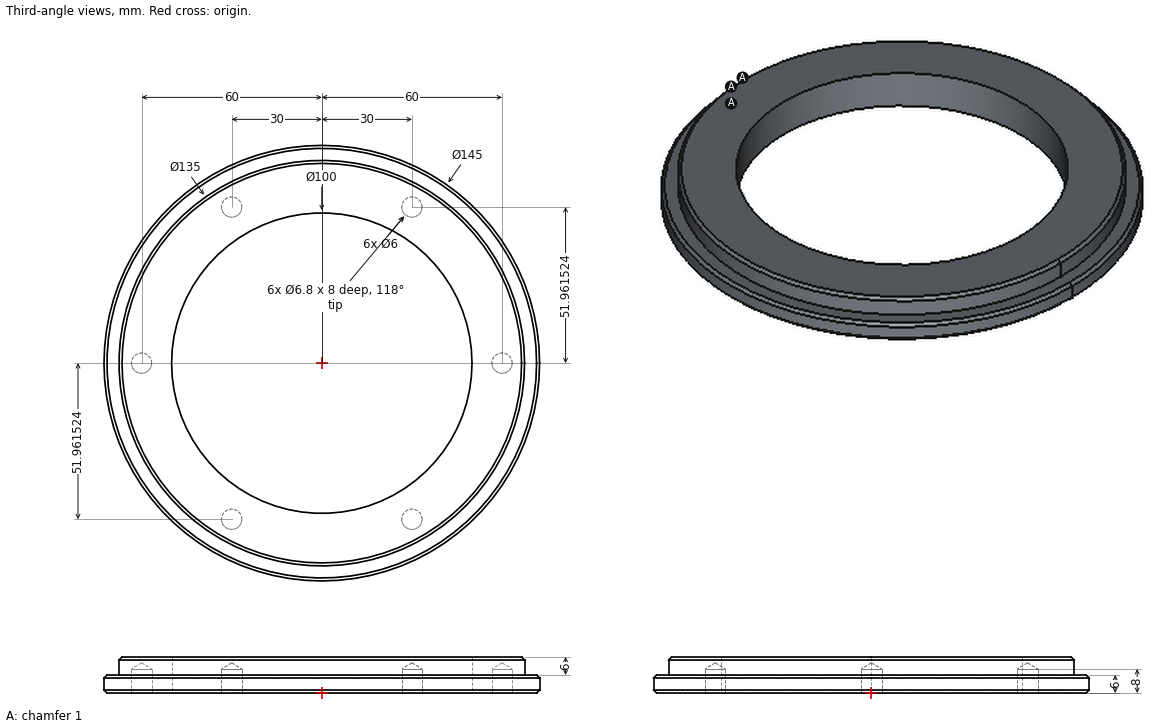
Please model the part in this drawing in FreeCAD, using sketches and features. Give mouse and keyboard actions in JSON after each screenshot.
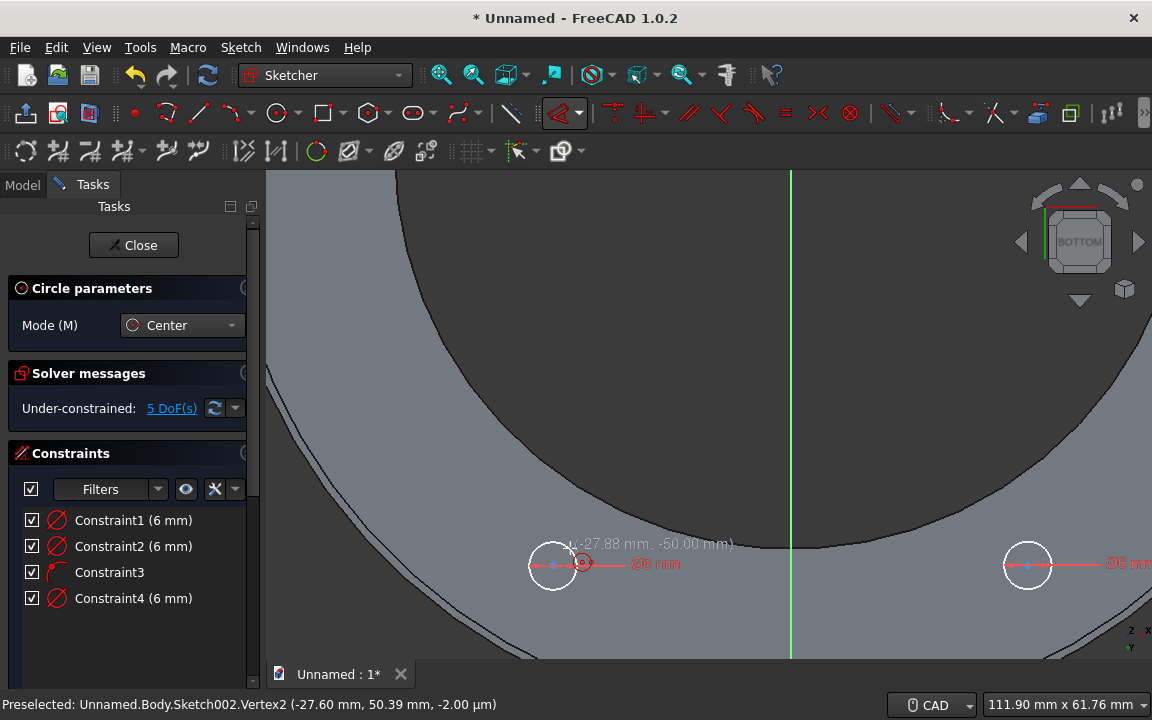
{"action": "scroll", "coordinate": [553, 567], "scroll_direction": "down", "scroll_amount": 5}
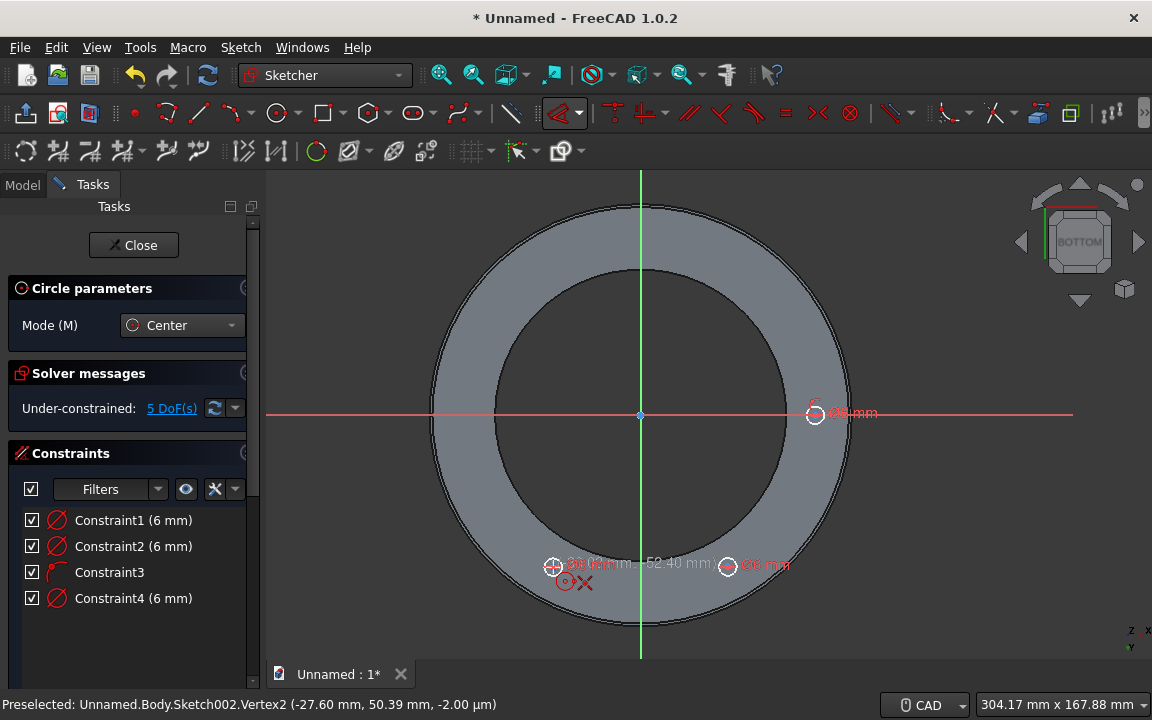
{"action": "scroll", "coordinate": [466, 415], "scroll_direction": "up", "scroll_amount": 5}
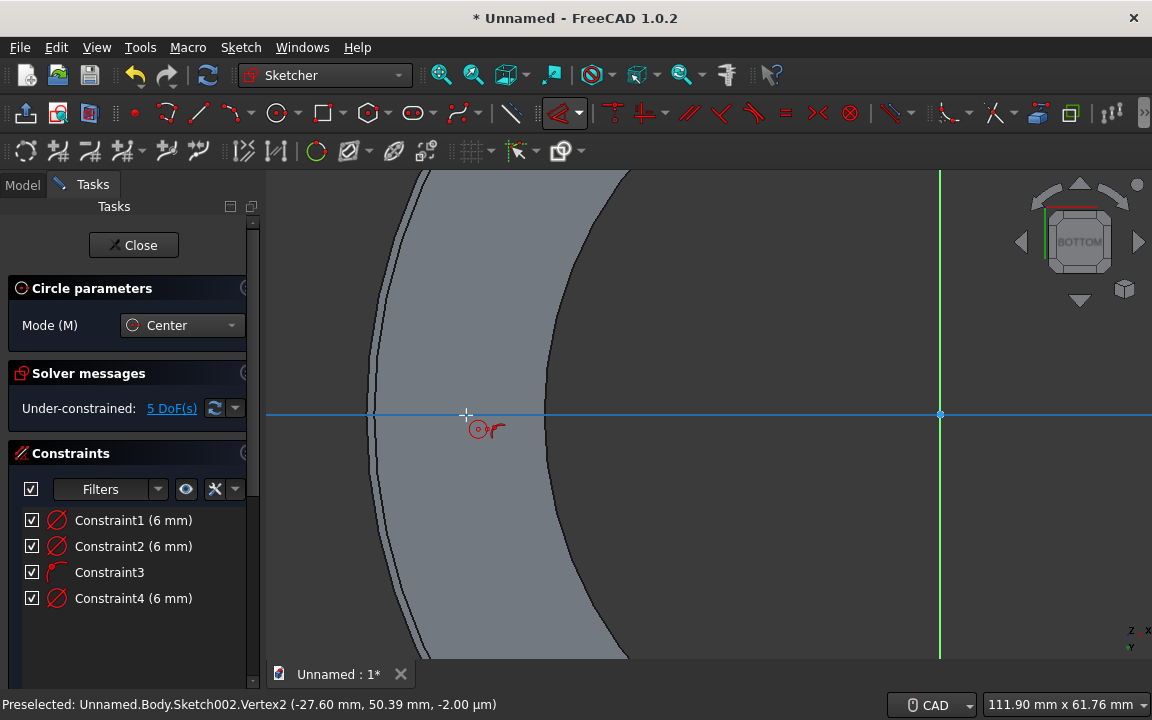
{"action": "left_click", "coordinate": [465, 415]}
{"action": "mouse_move", "coordinate": [482, 398]}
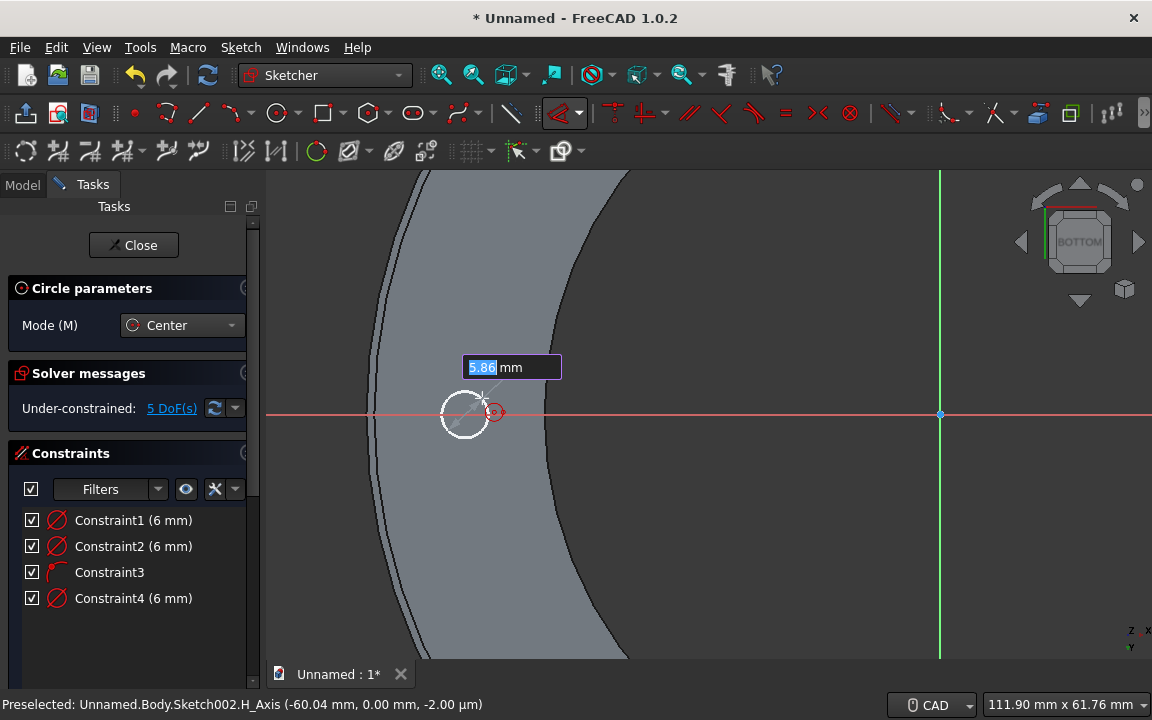
{"action": "type", "text": "6"}
{"action": "key", "text": "Return"}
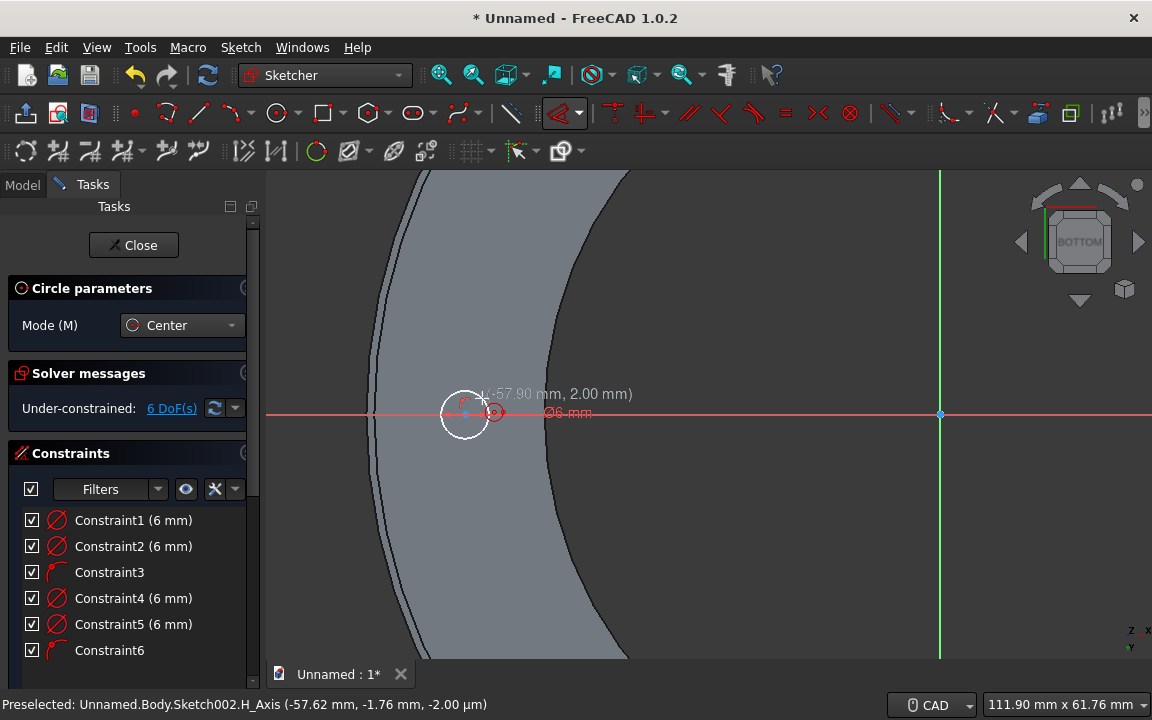
{"action": "scroll", "coordinate": [466, 414], "scroll_direction": "down", "scroll_amount": 5}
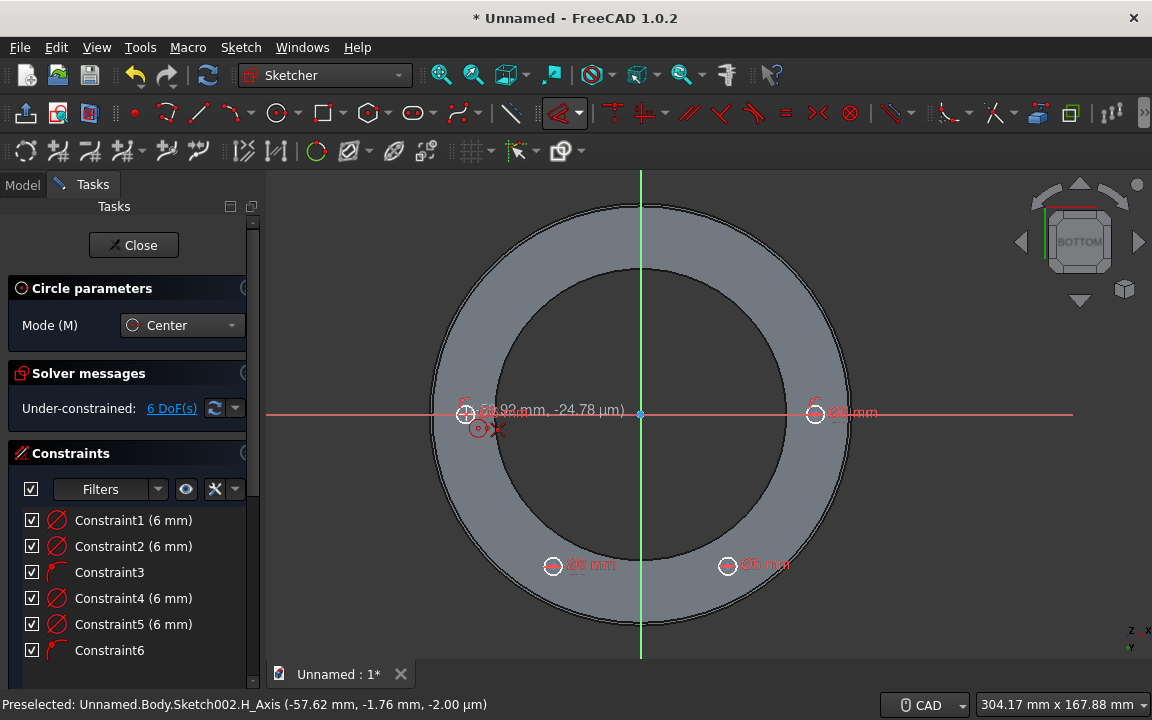
{"action": "scroll", "coordinate": [553, 263], "scroll_direction": "up", "scroll_amount": 5}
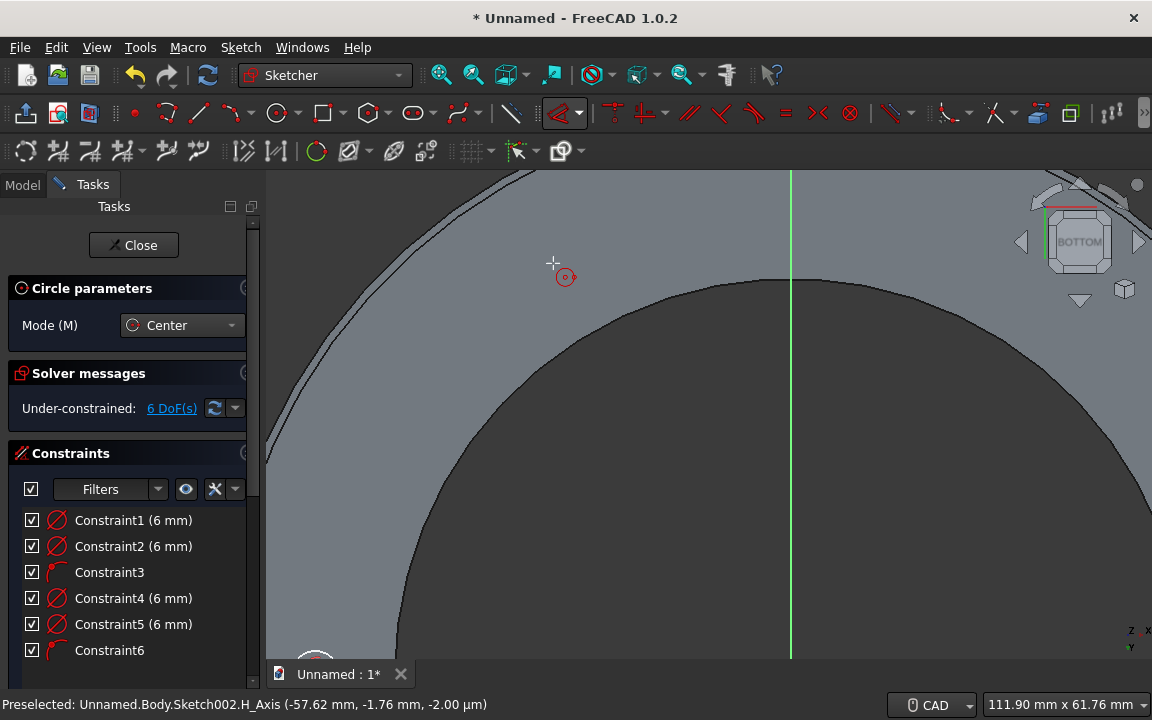
{"action": "left_click", "coordinate": [553, 263]}
{"action": "mouse_move", "coordinate": [570, 247]}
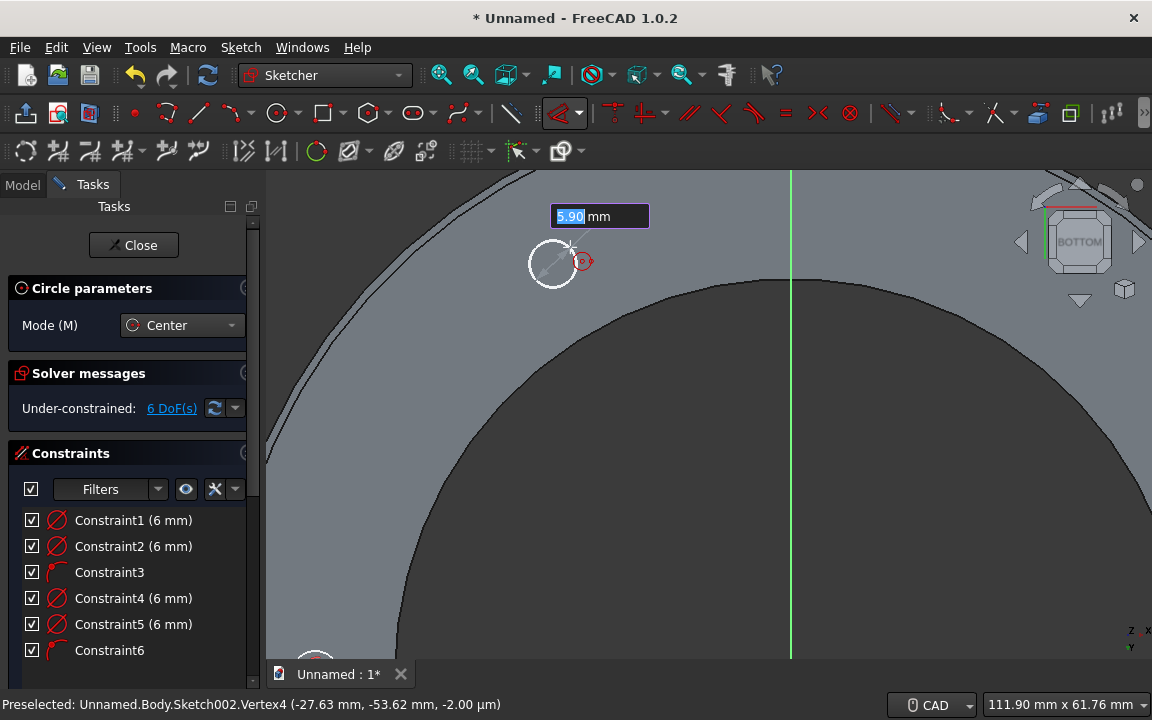
{"action": "type", "text": "6"}
{"action": "key", "text": "Return"}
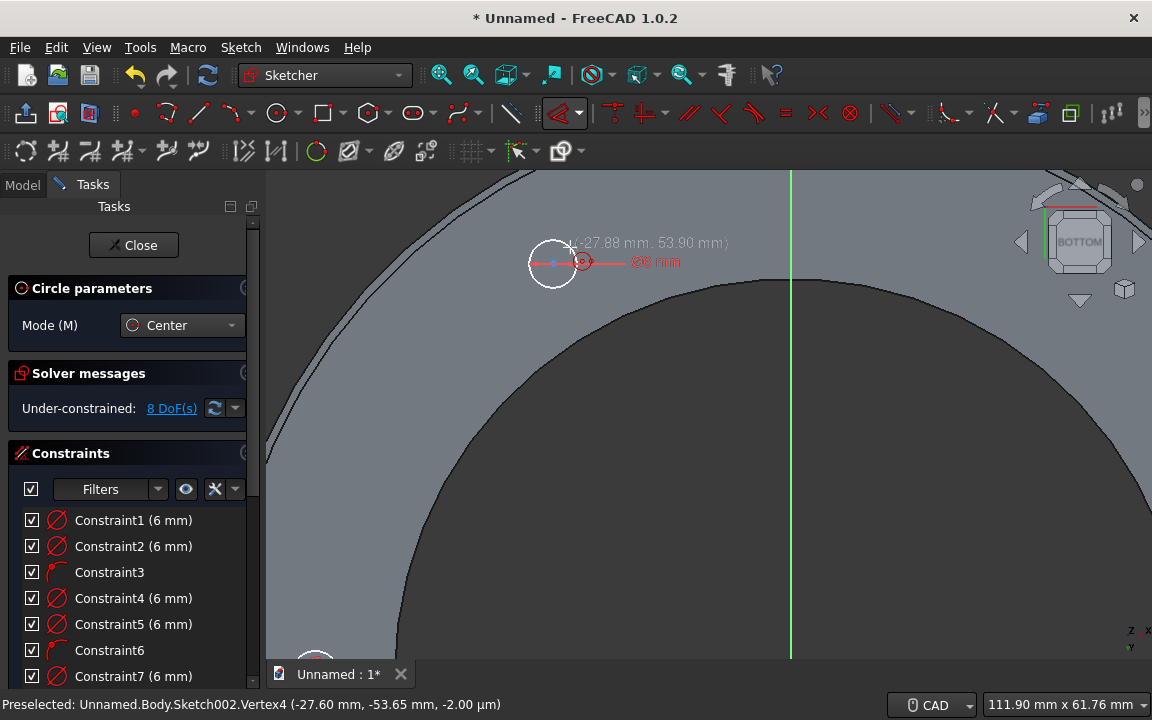
{"action": "scroll", "coordinate": [553, 263], "scroll_direction": "down", "scroll_amount": 5}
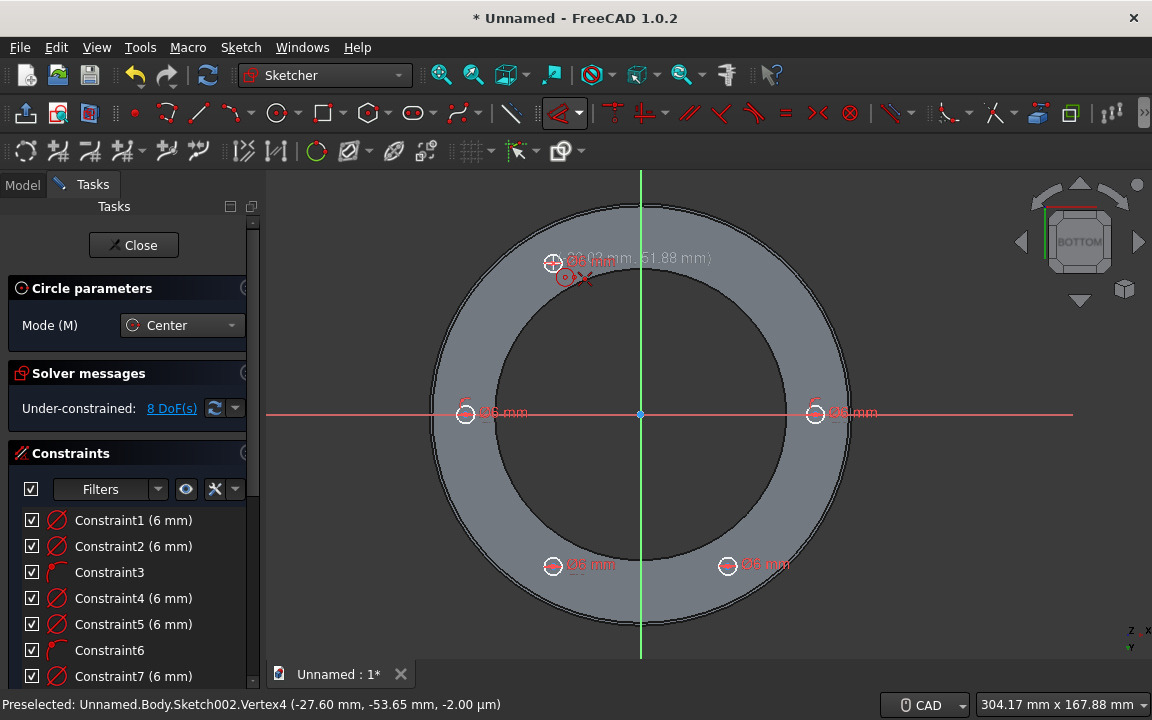
{"action": "scroll", "coordinate": [728, 263], "scroll_direction": "up", "scroll_amount": 5}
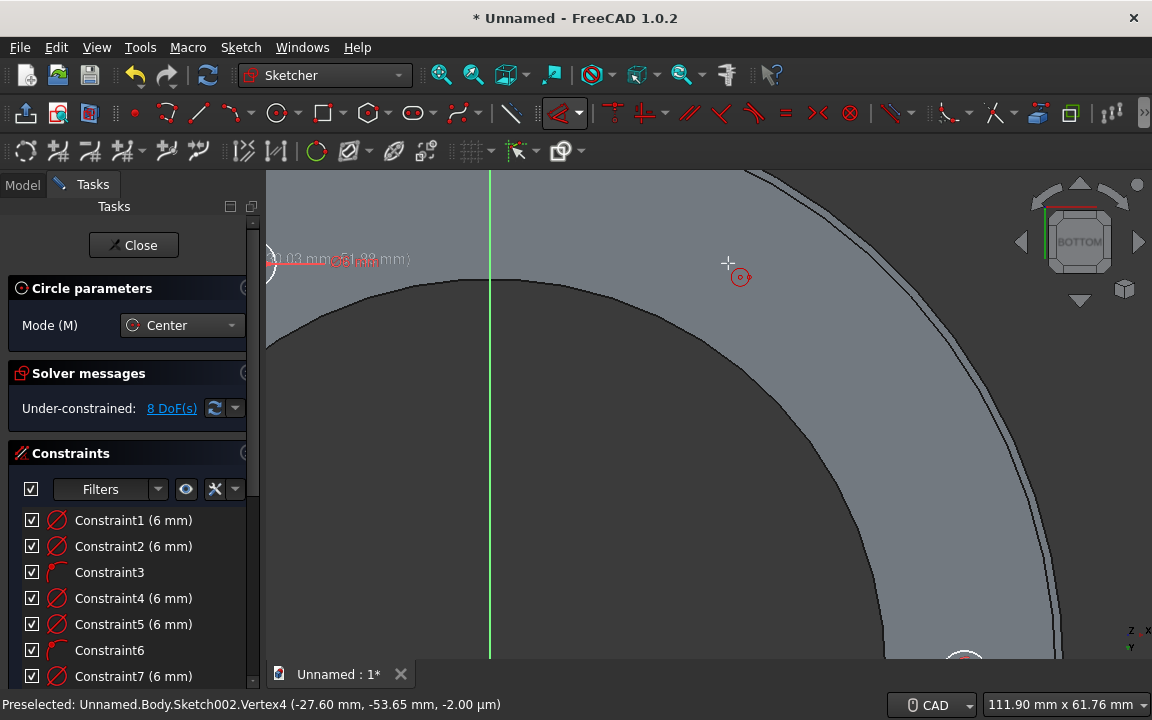
{"action": "left_click", "coordinate": [727, 263]}
{"action": "mouse_move", "coordinate": [744, 247]}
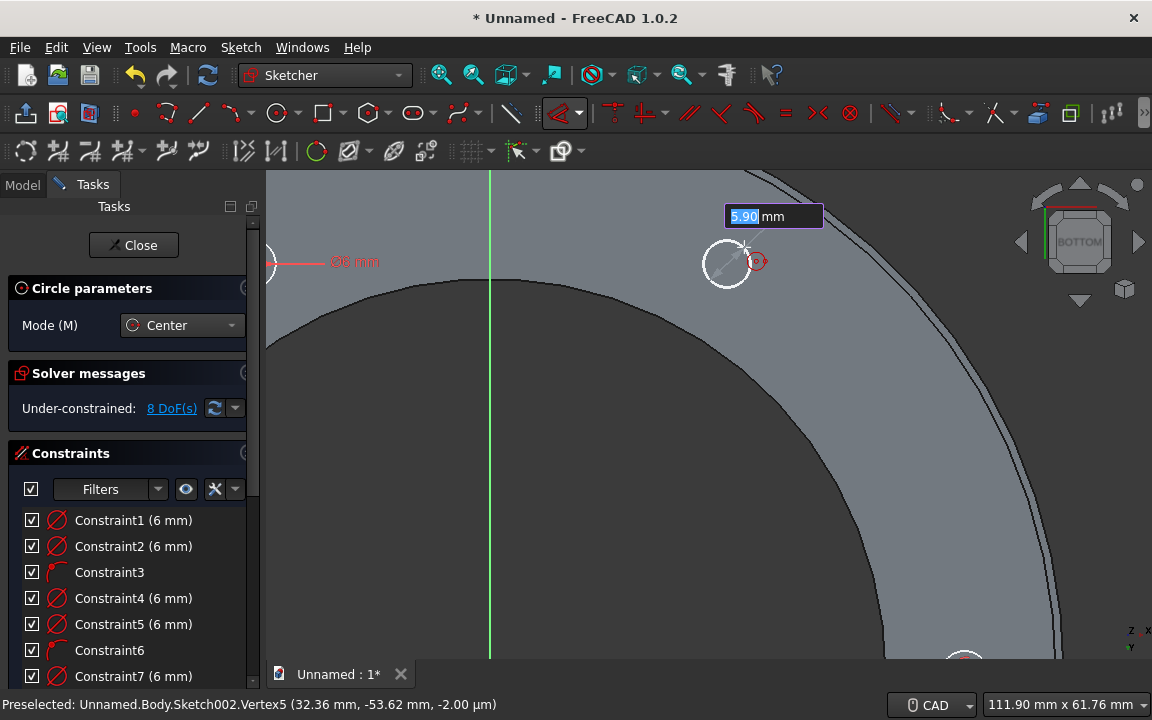
{"action": "type", "text": "6"}
{"action": "key", "text": "Return"}
{"action": "key", "text": "Escape"}